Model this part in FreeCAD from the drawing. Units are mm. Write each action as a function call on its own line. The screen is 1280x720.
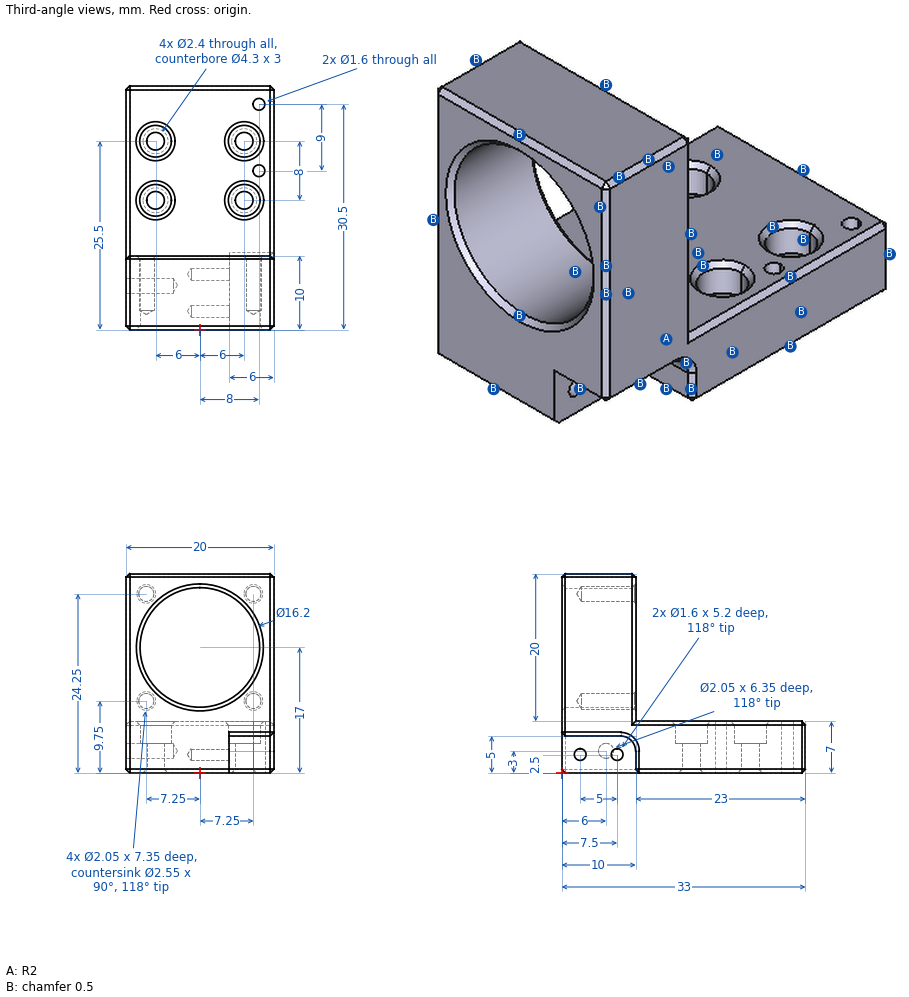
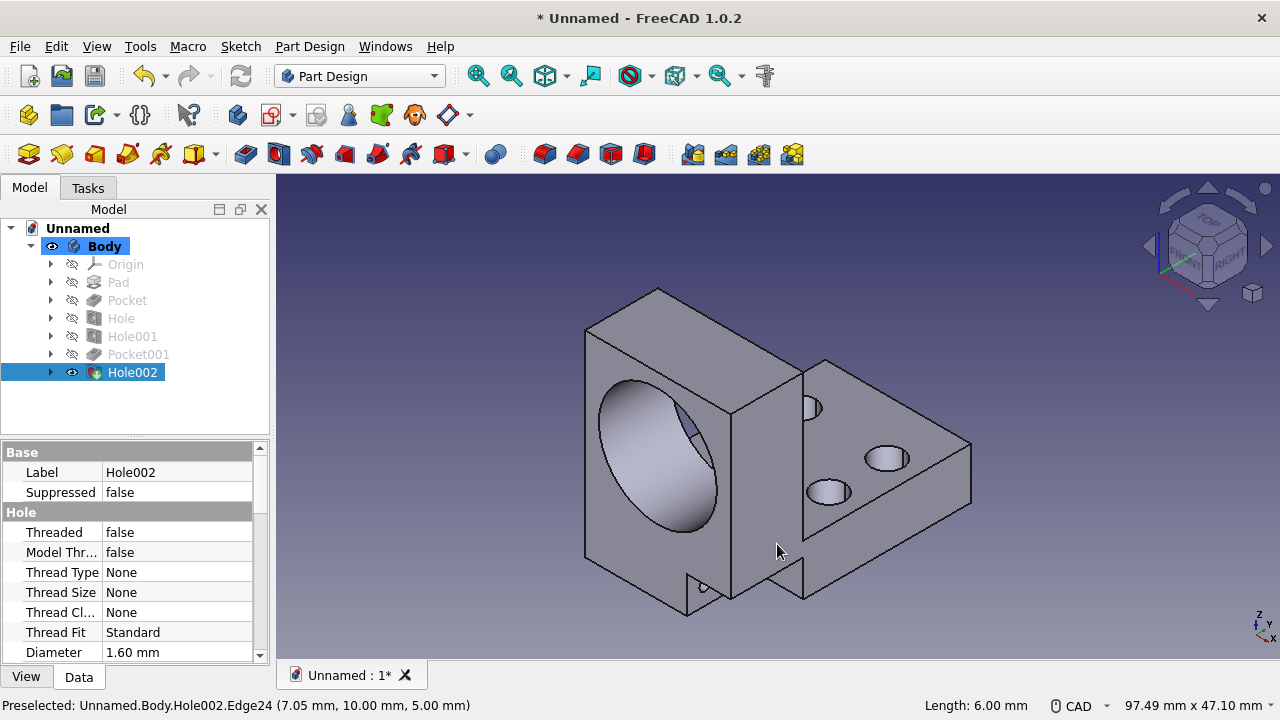
click(545, 154)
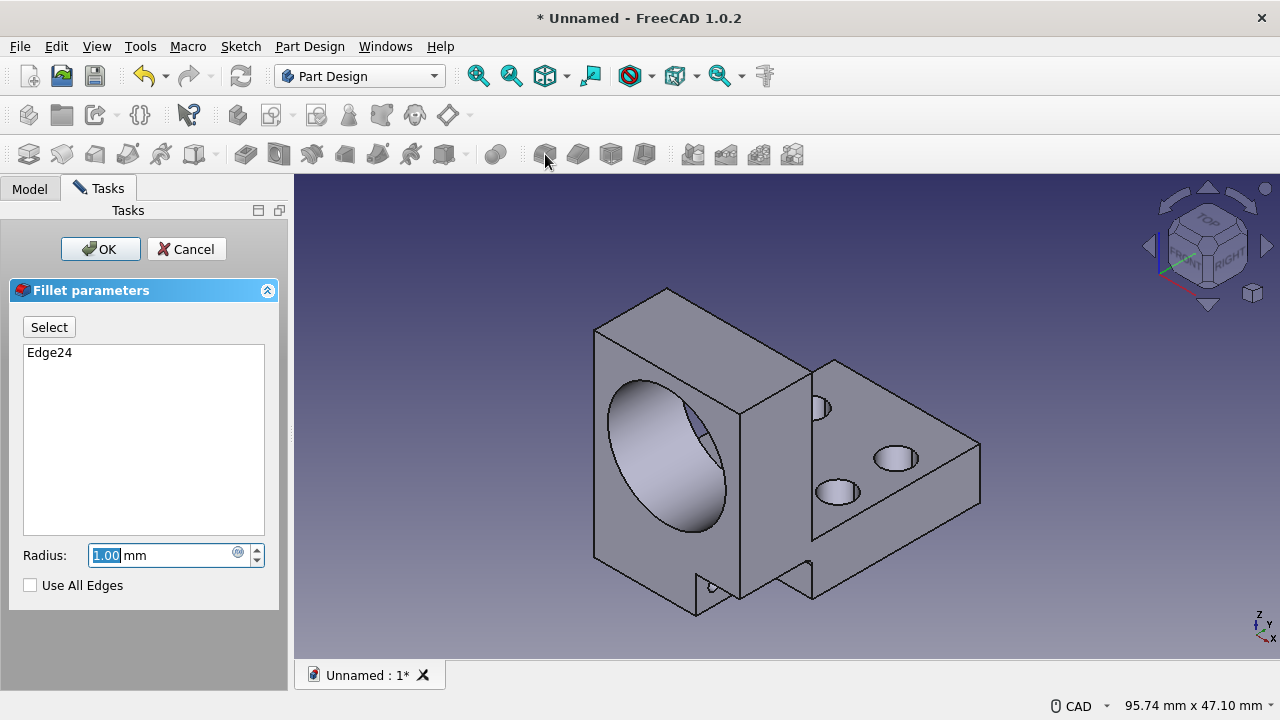
text(2)
key(Tab)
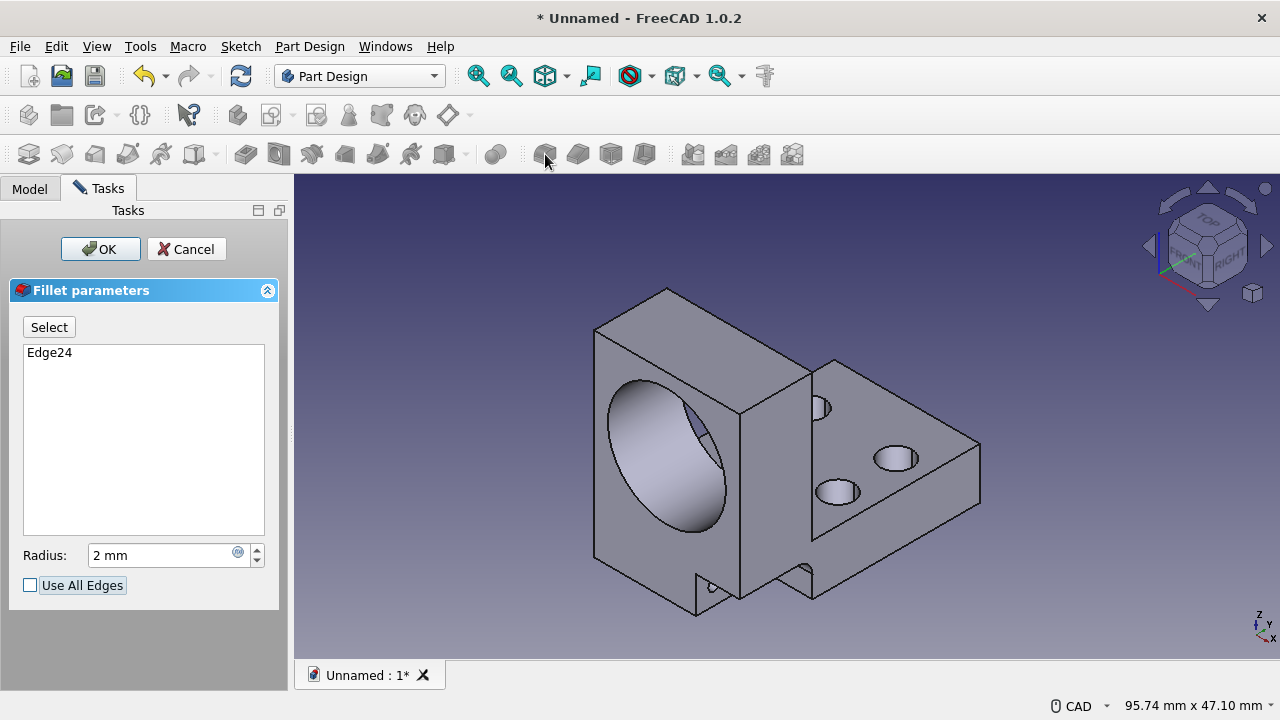
click(101, 249)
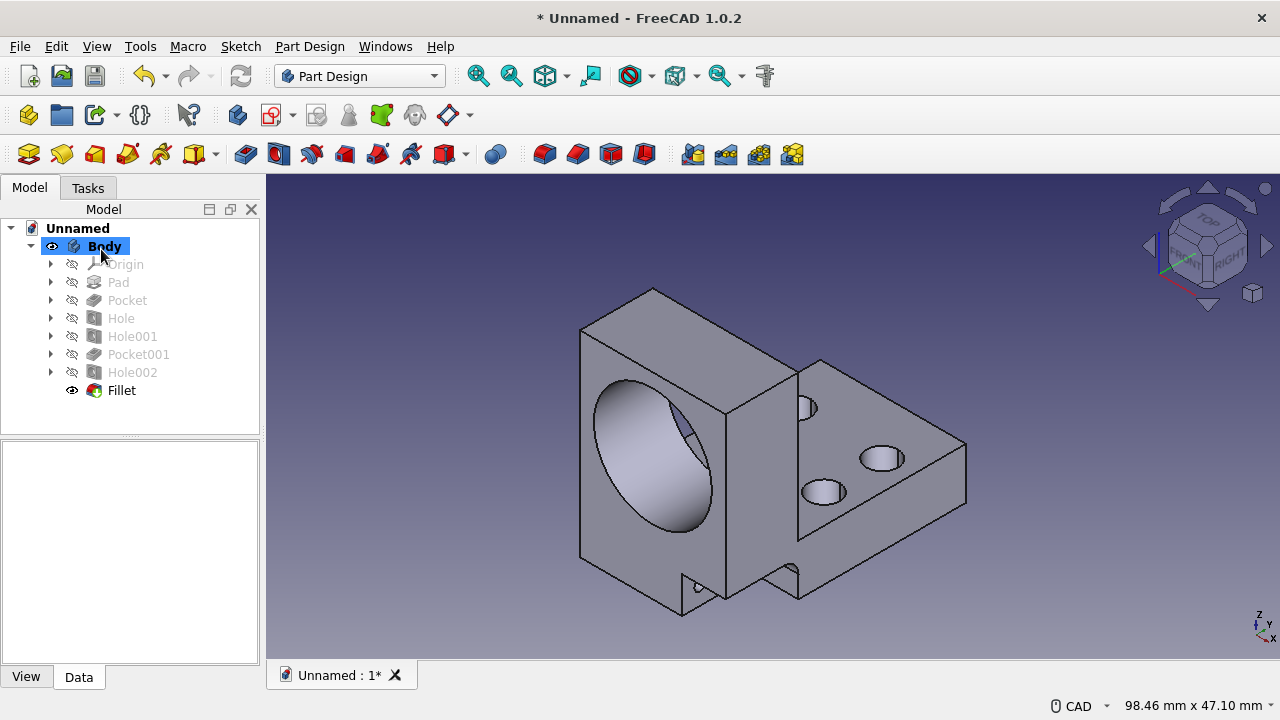
click(777, 530)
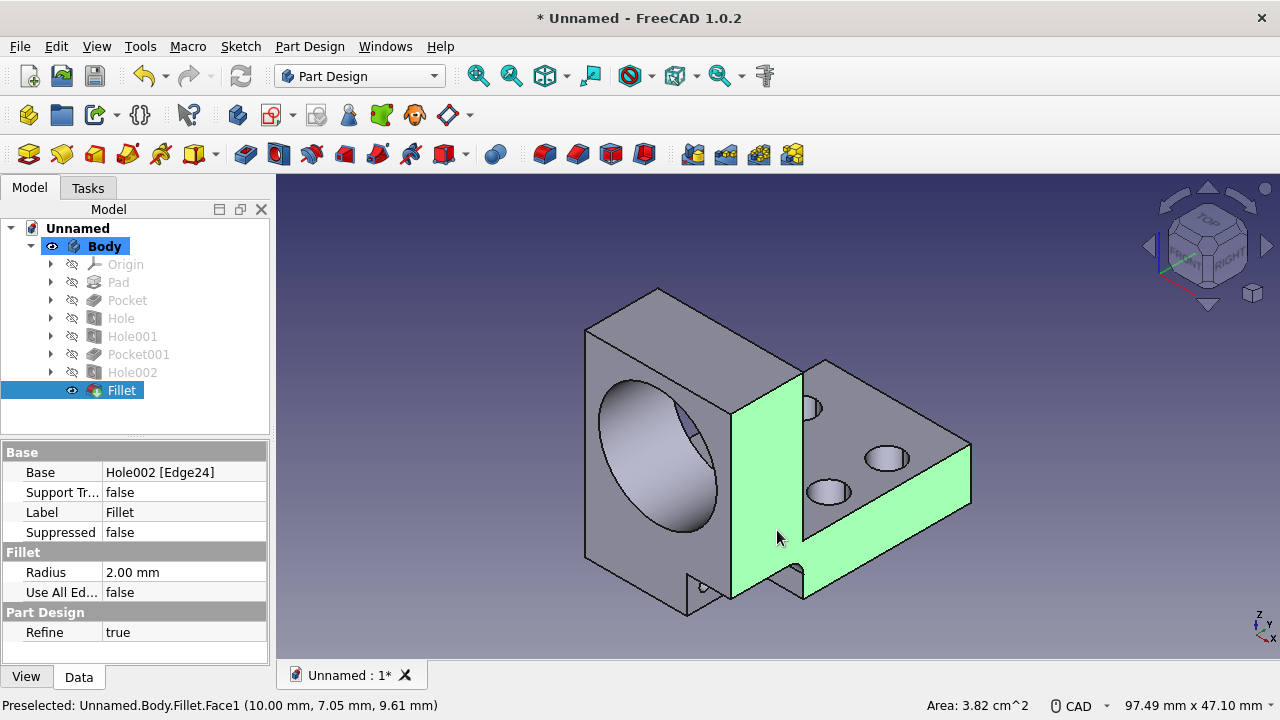
click(658, 371, ctrl)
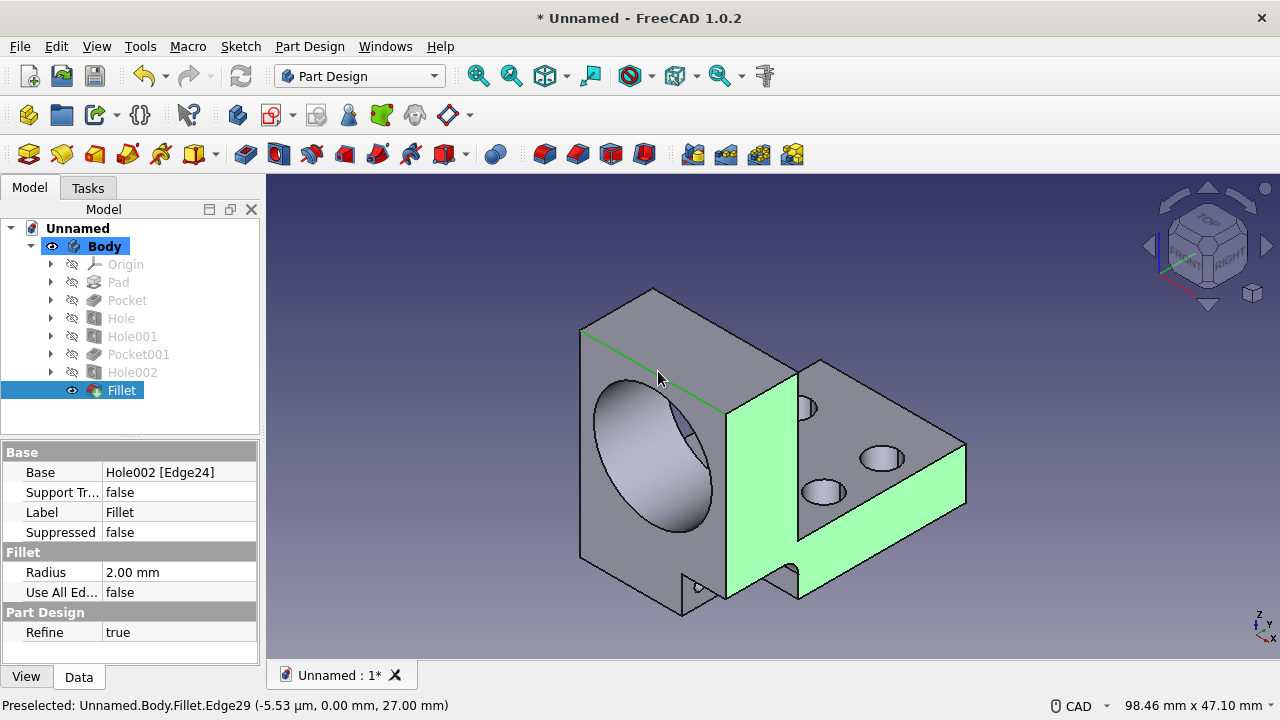
click(653, 524, ctrl)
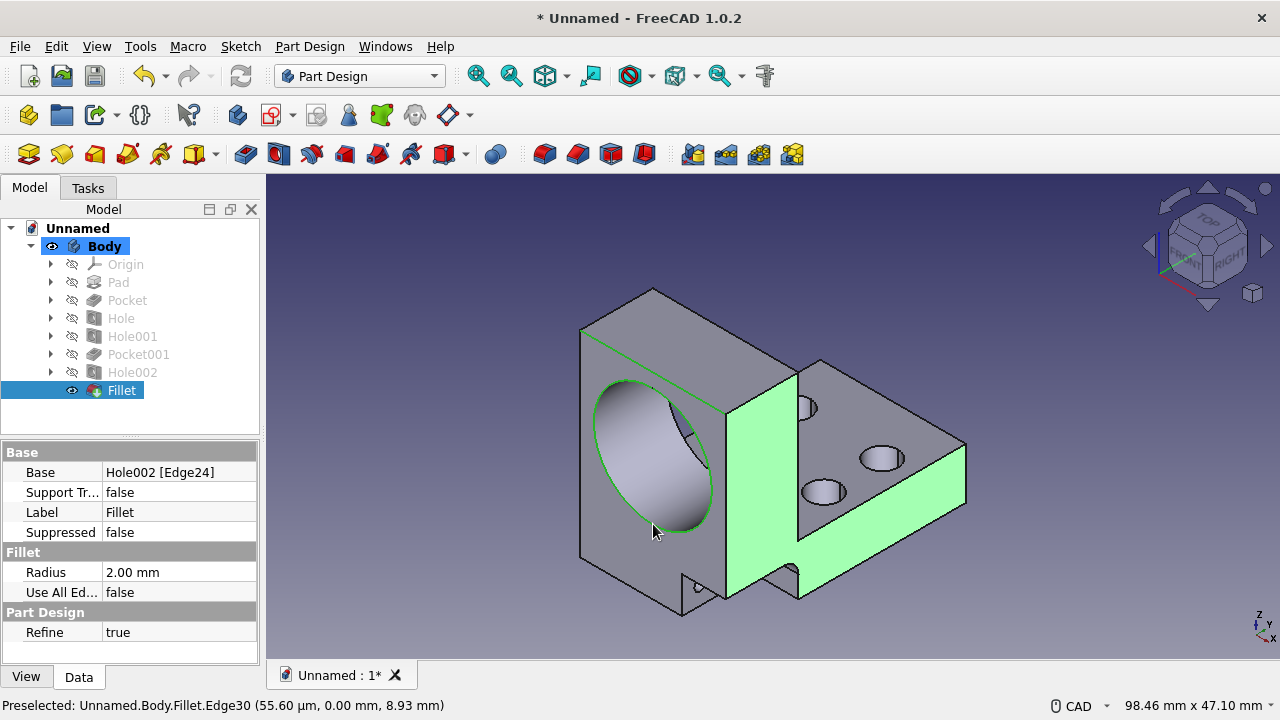
click(814, 480, ctrl)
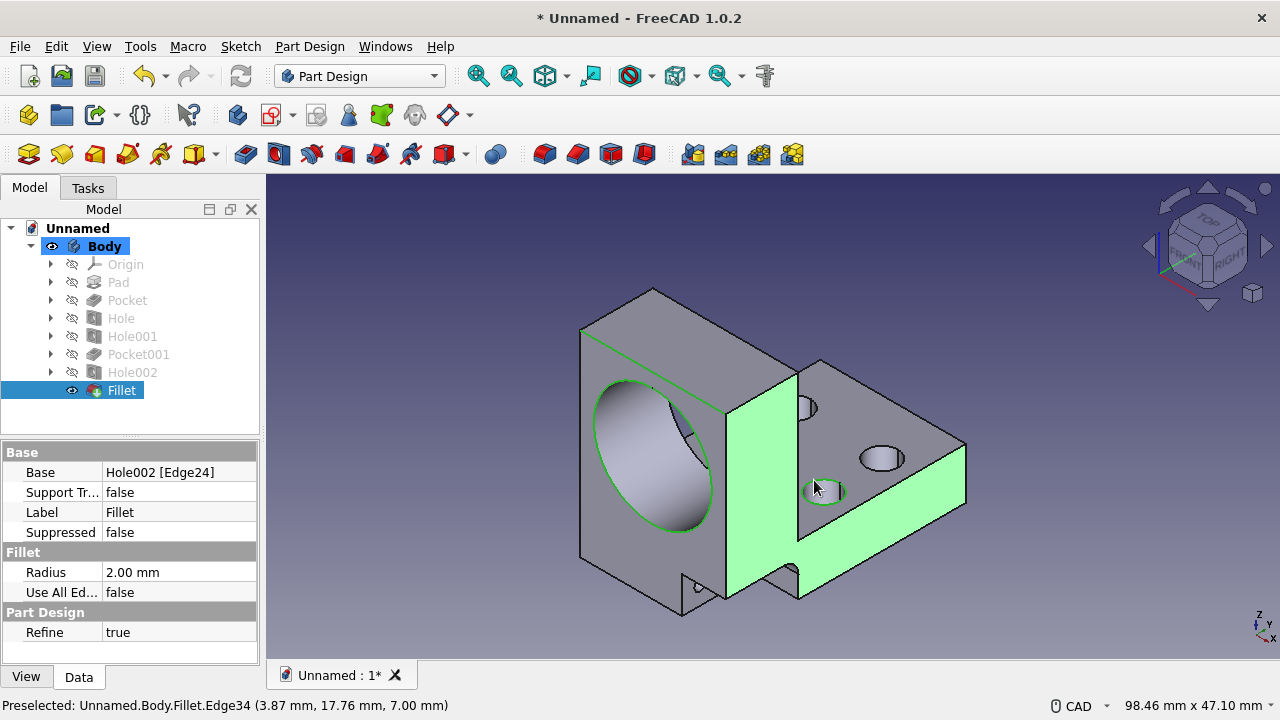
click(860, 460, ctrl)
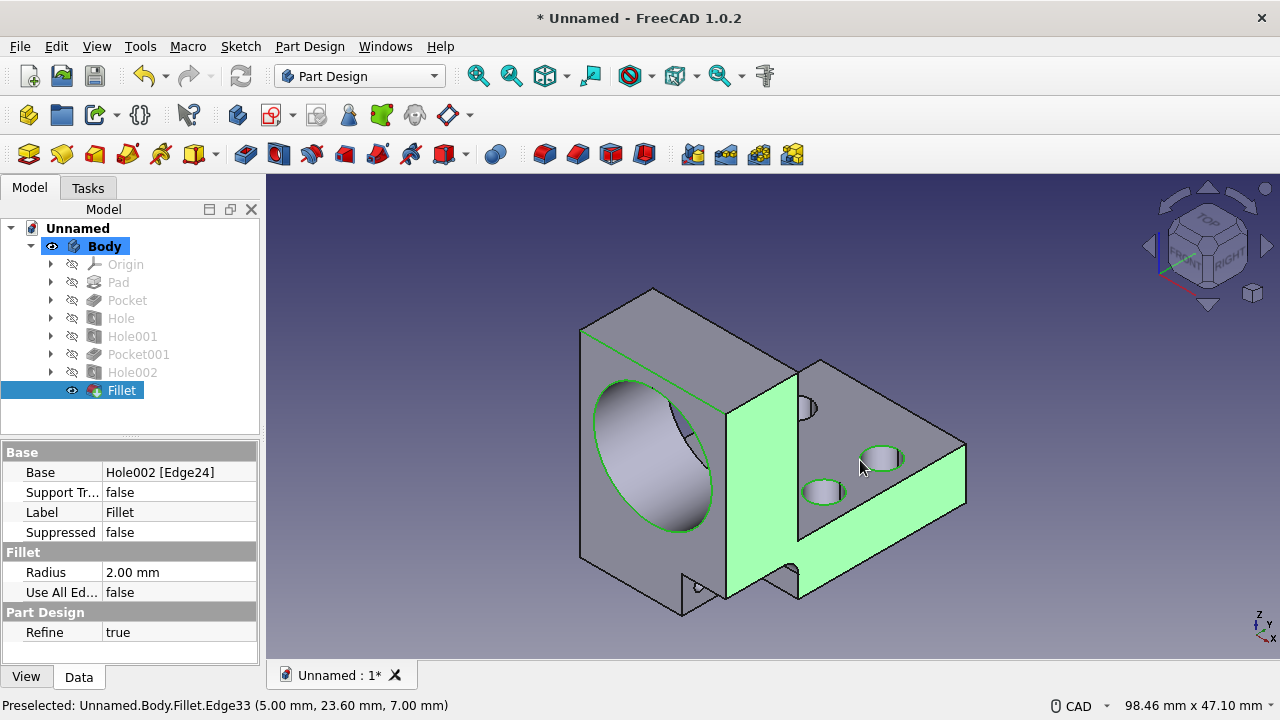
click(815, 413, ctrl)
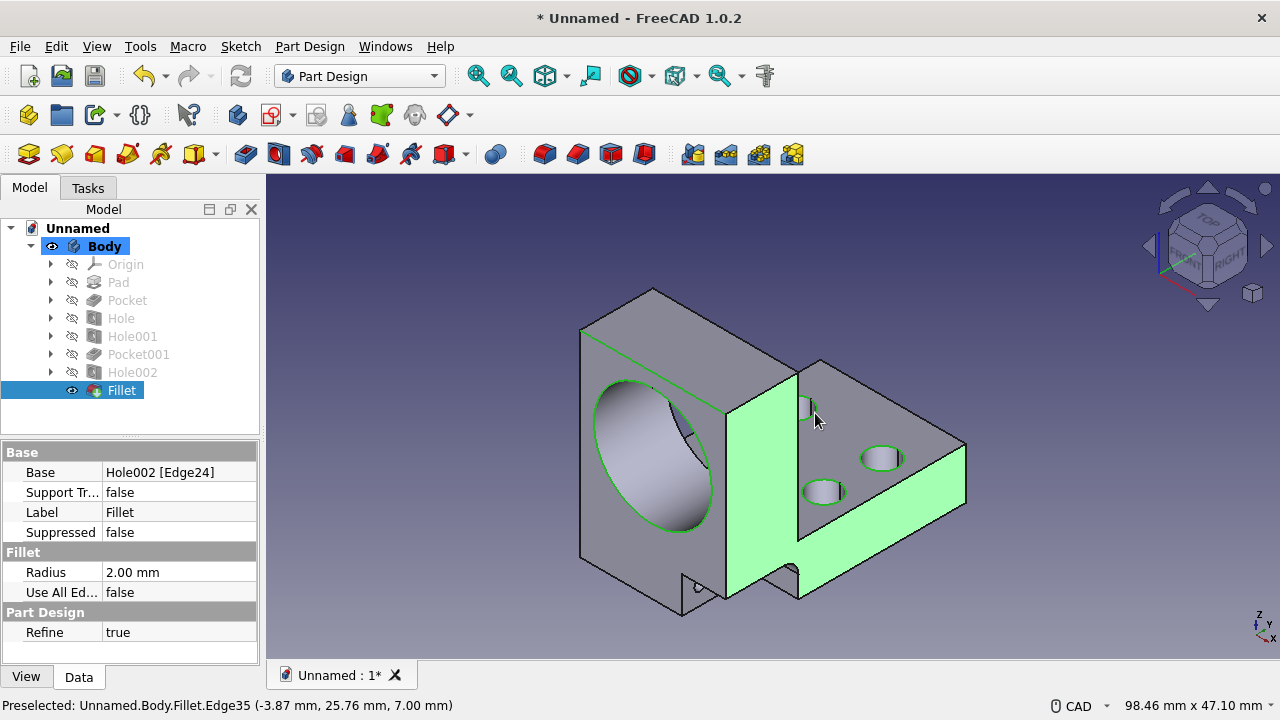
key(2)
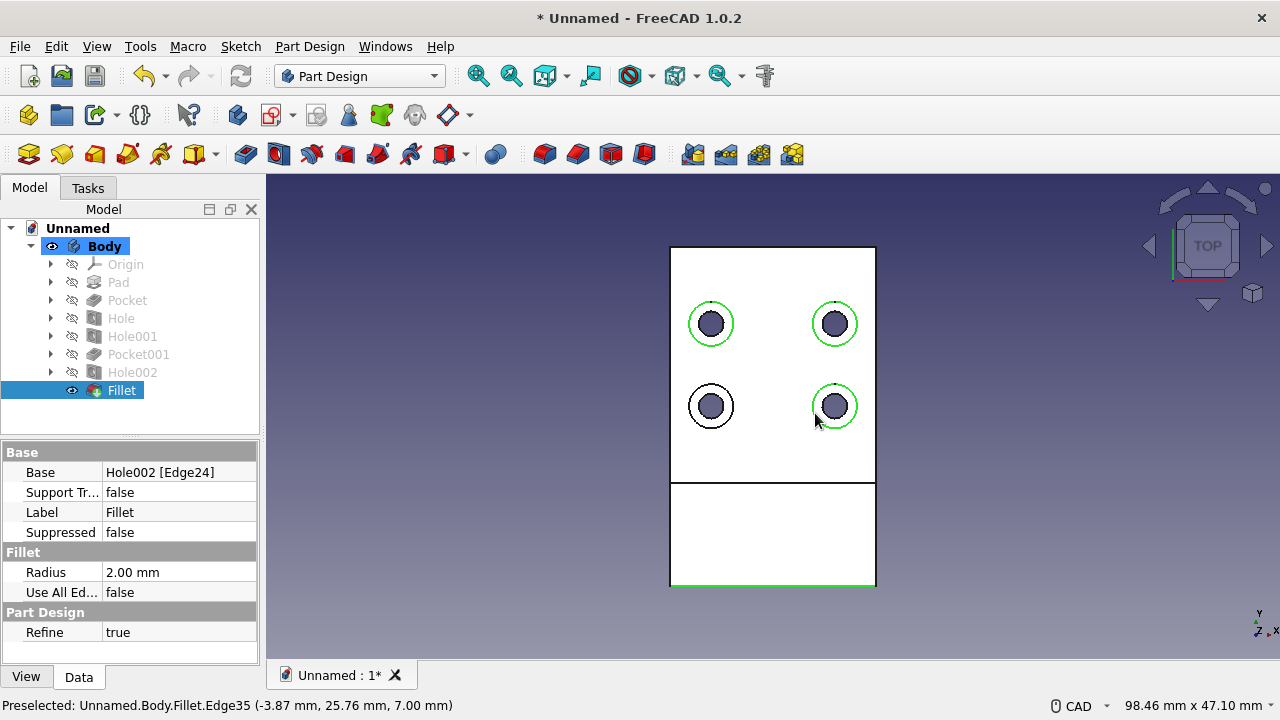
click(773, 482, ctrl)